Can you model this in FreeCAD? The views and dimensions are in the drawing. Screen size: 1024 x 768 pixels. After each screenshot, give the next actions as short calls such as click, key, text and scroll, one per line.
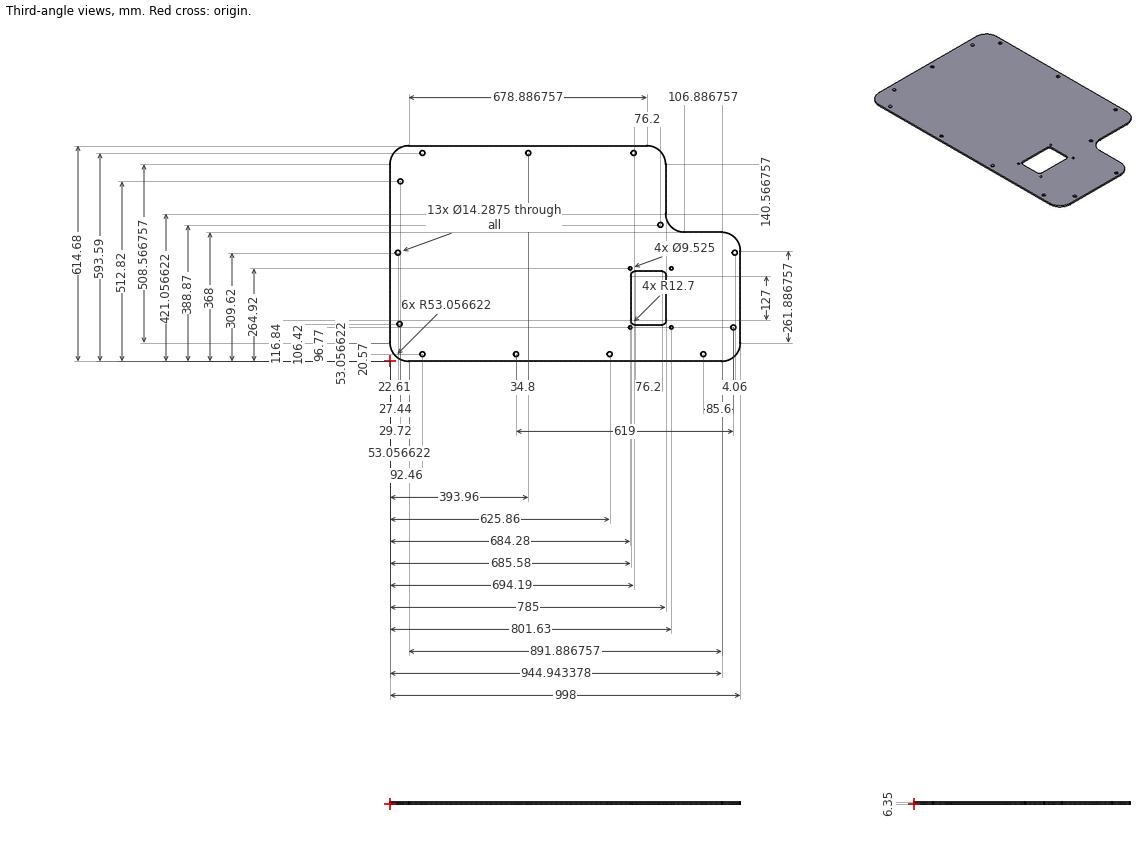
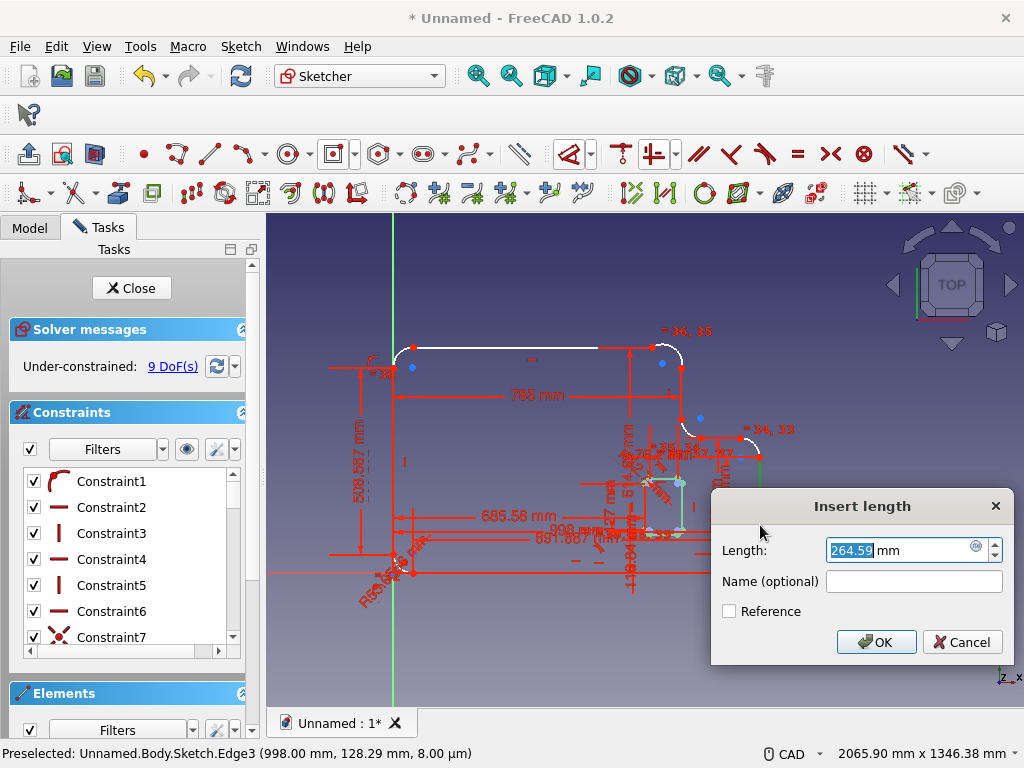
text(261.886757)
key(Return)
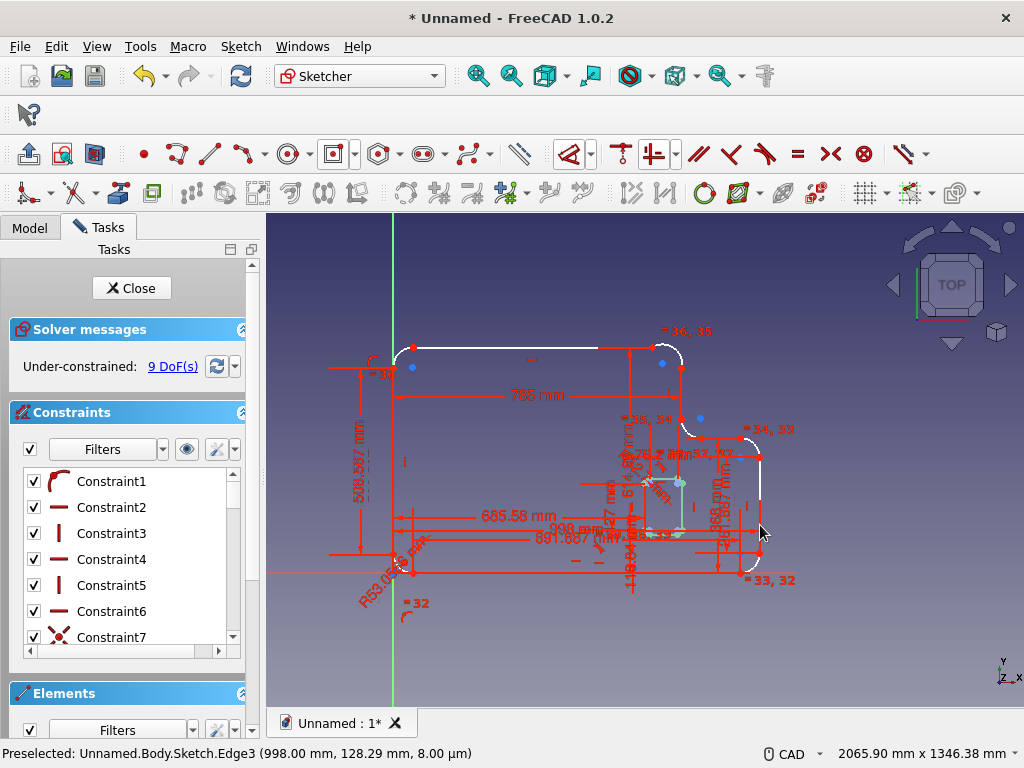
click(728, 438)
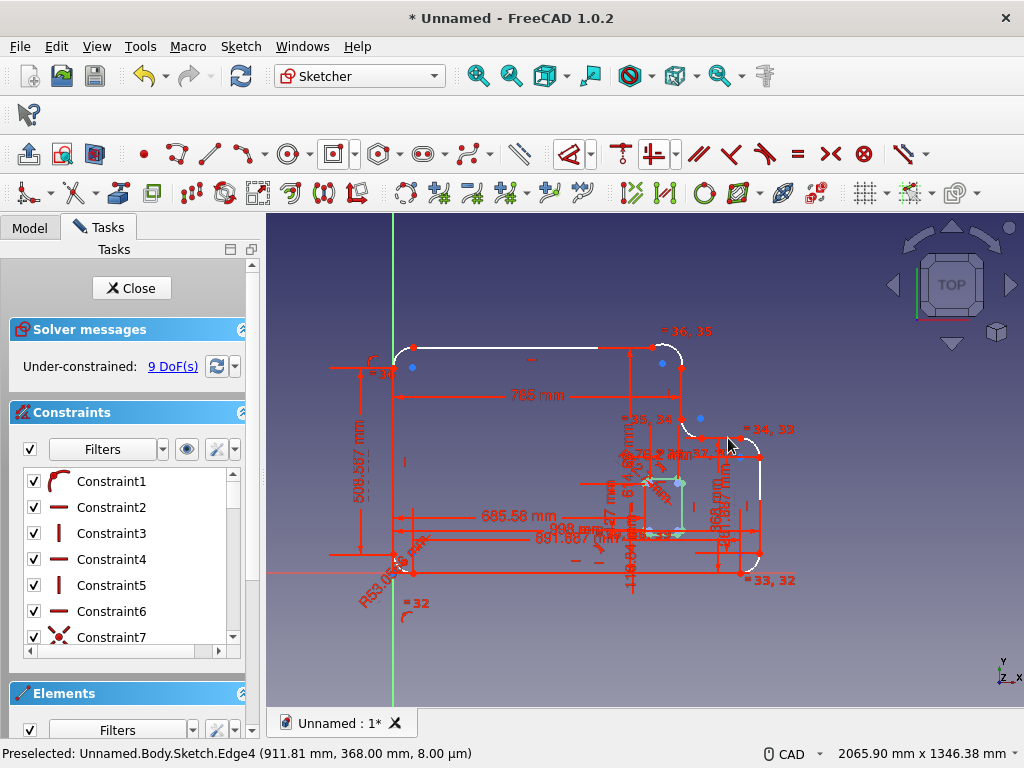
click(590, 154)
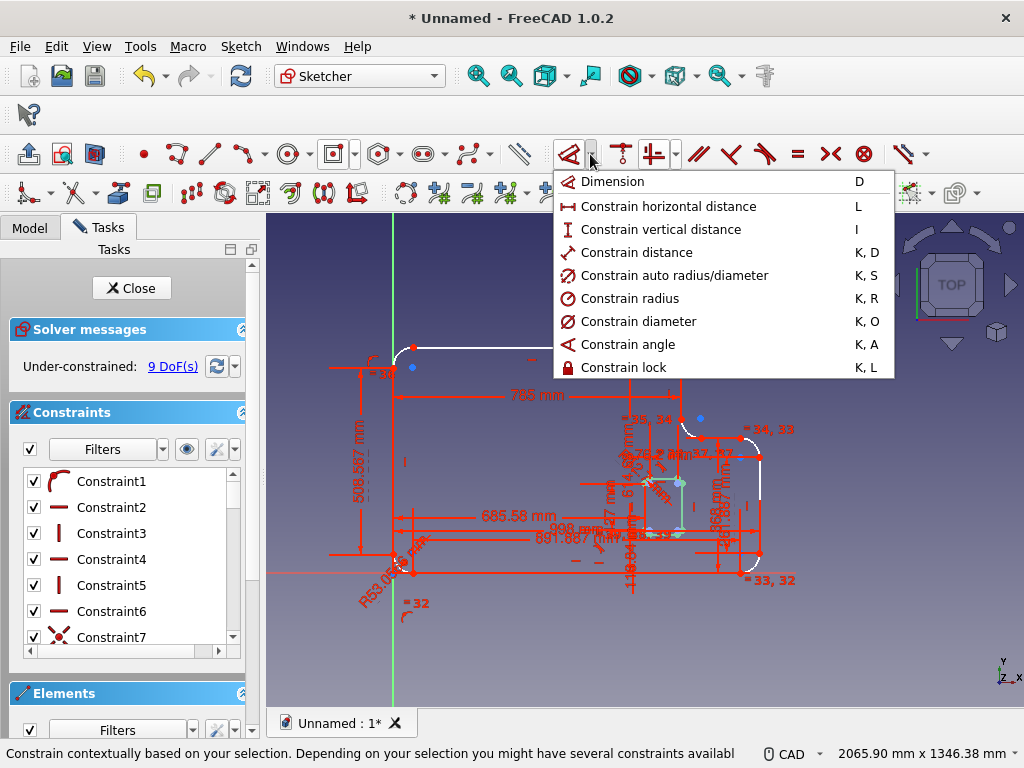
click(724, 206)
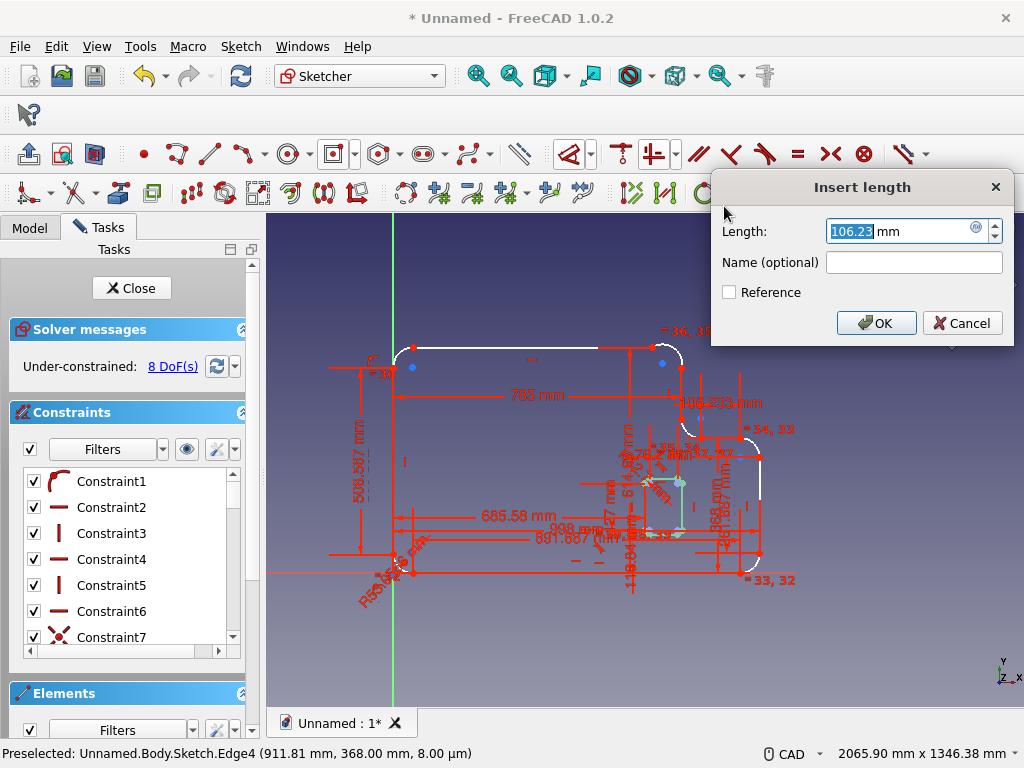
text(106.886757)
key(Return)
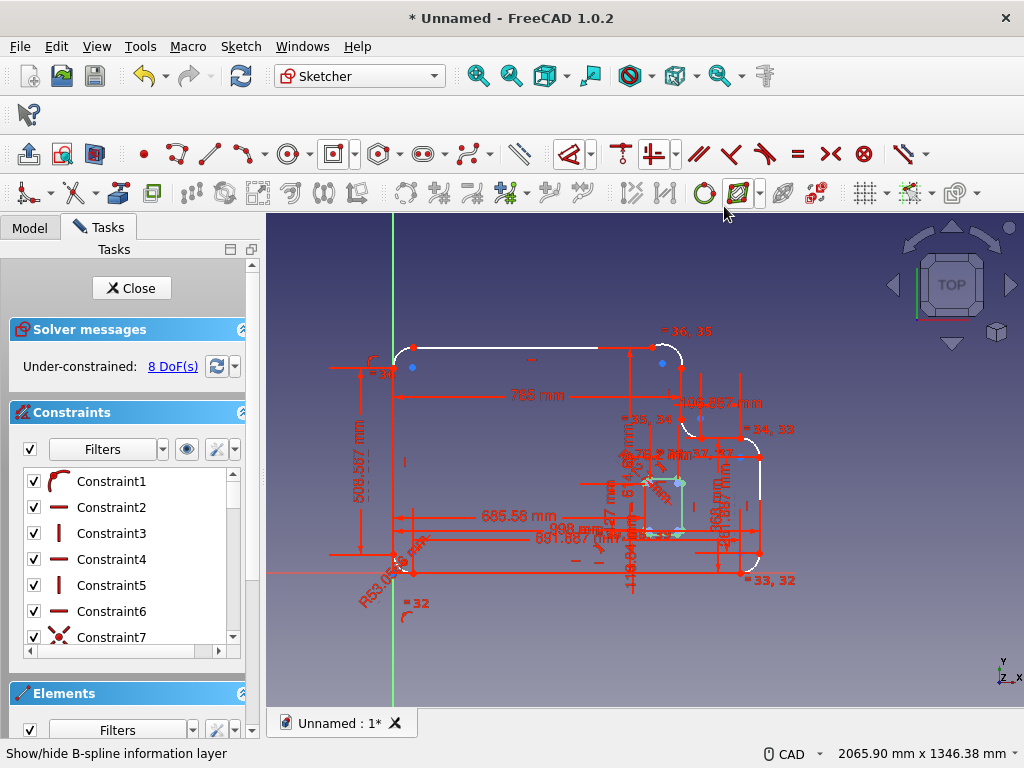
click(681, 384)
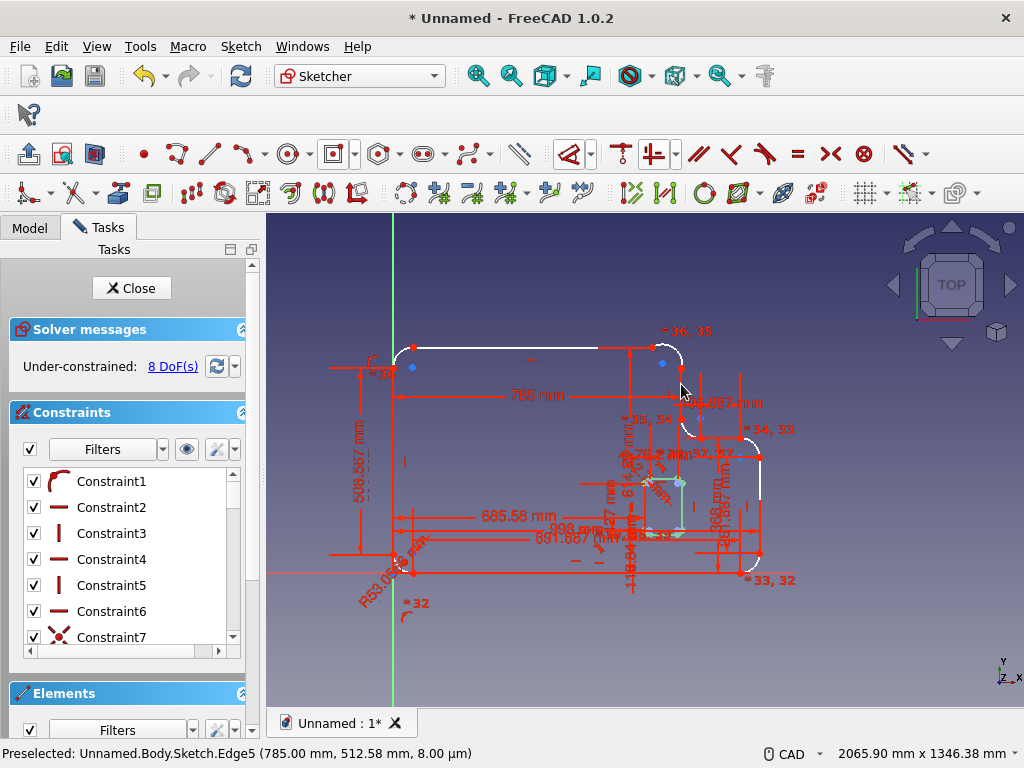
key(i)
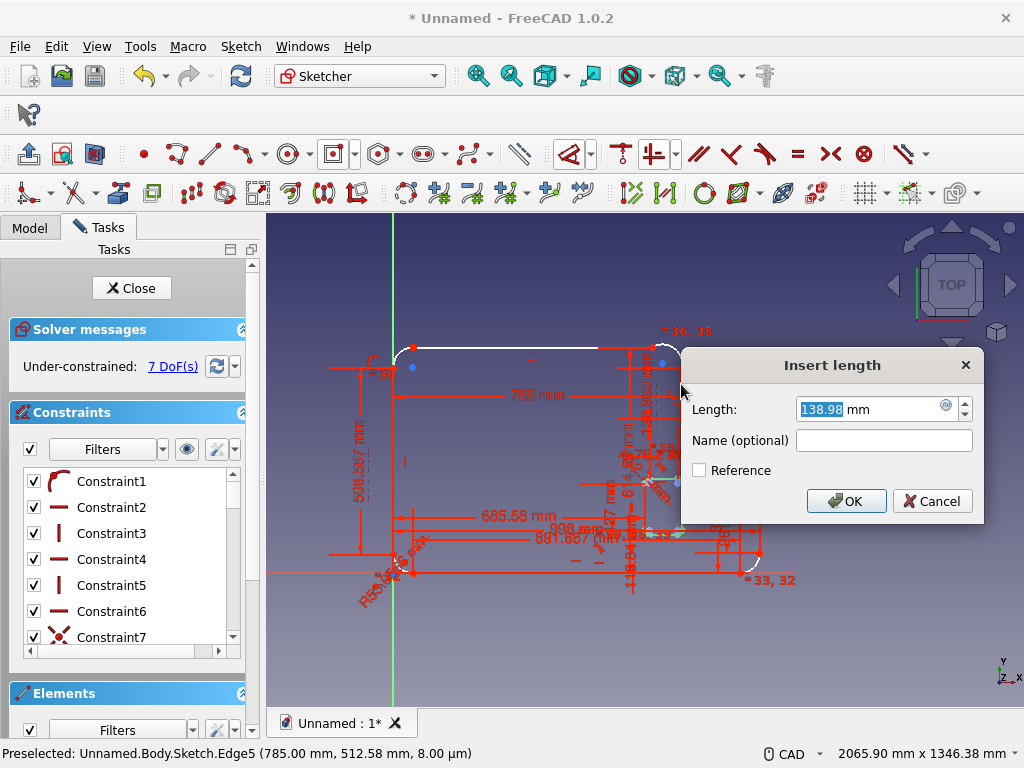
text(140.566757)
key(Return)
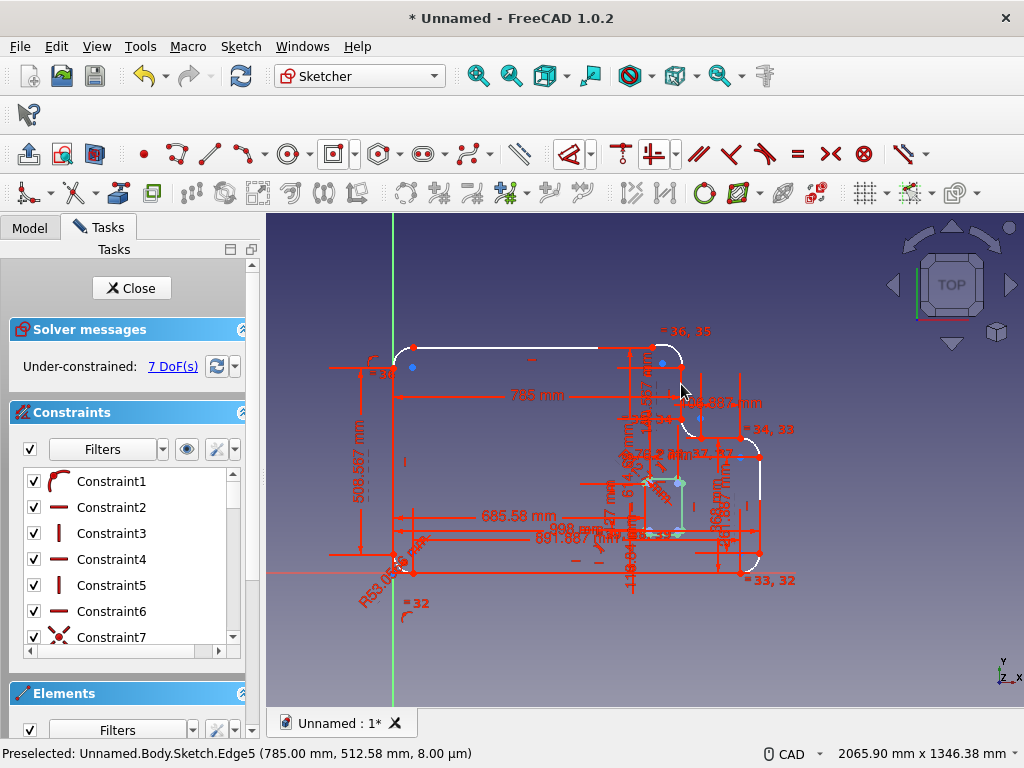
click(580, 348)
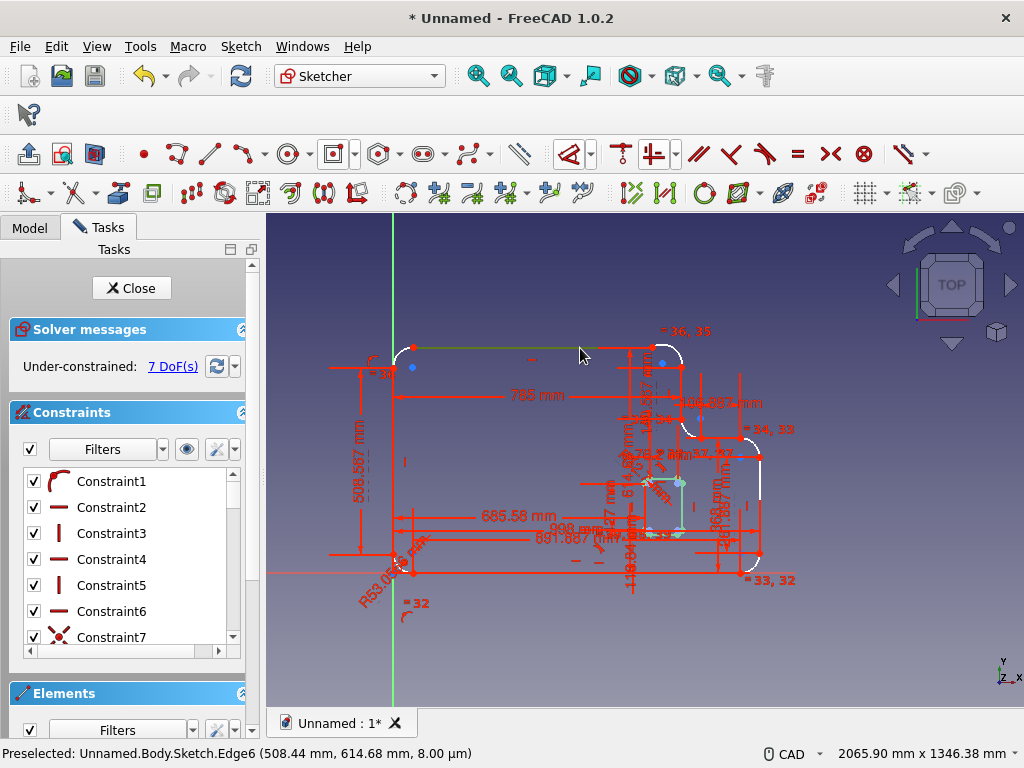
click(590, 154)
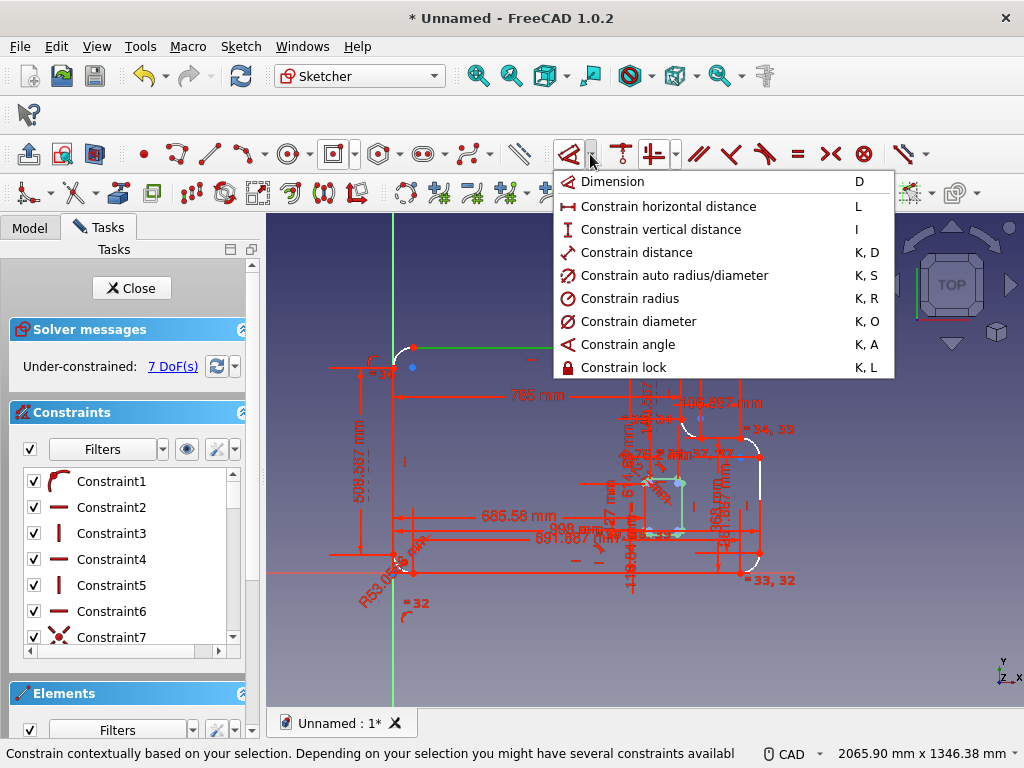
click(724, 206)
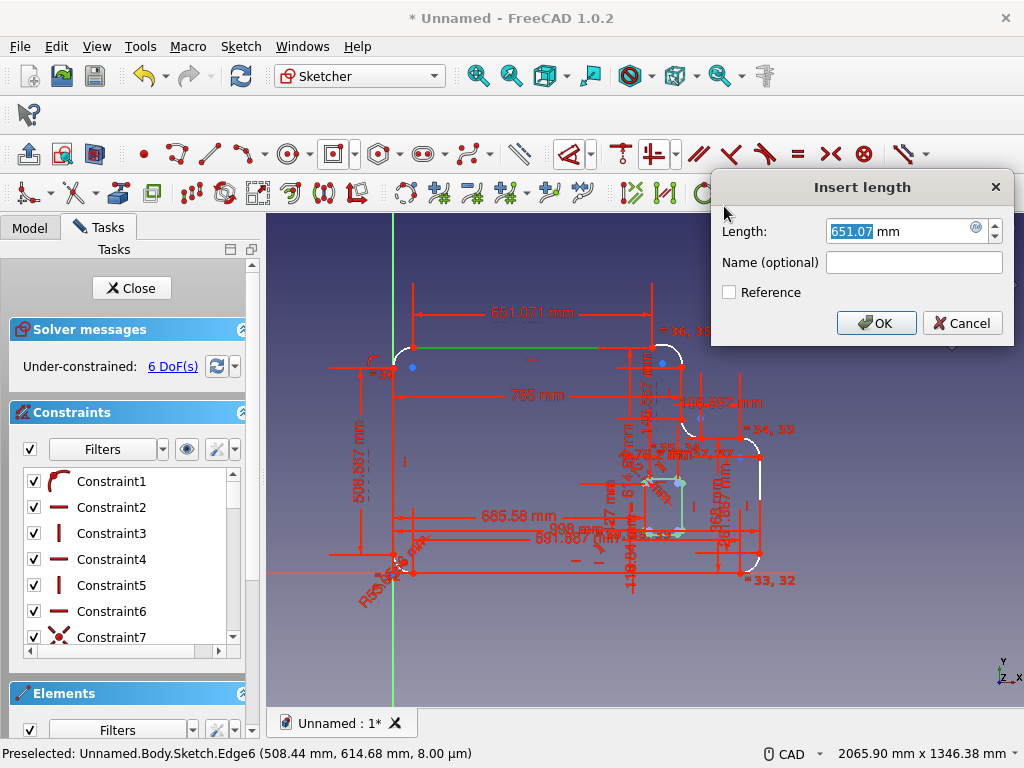
text(678.886757)
key(Return)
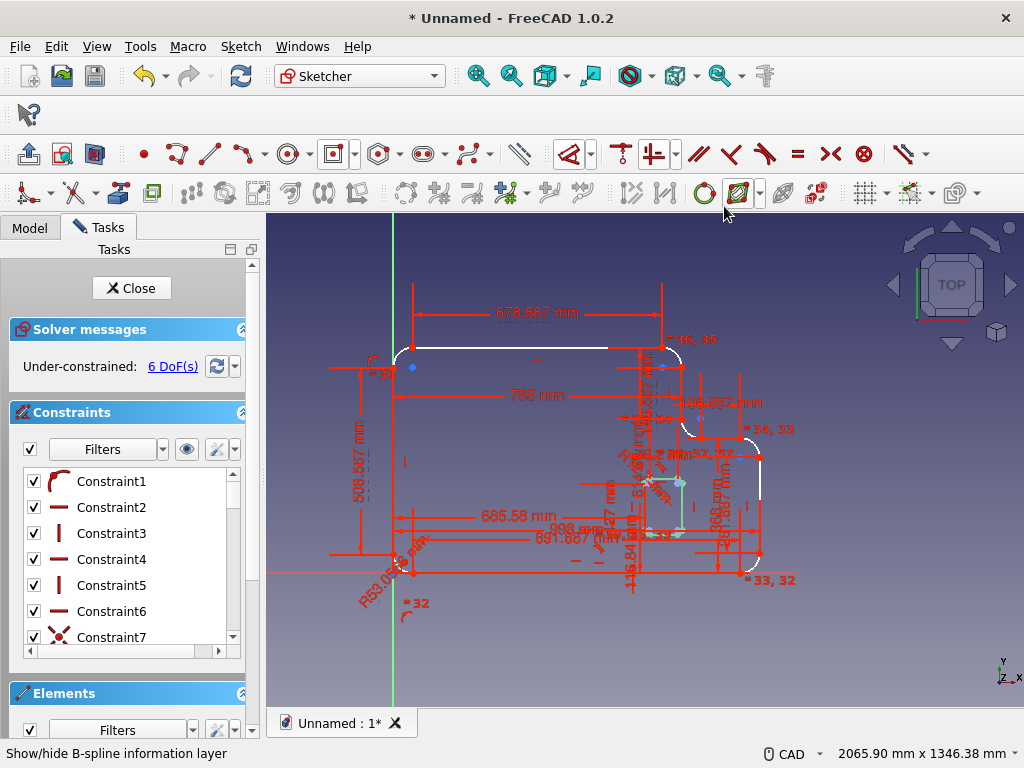
scroll(393, 555, up, 4)